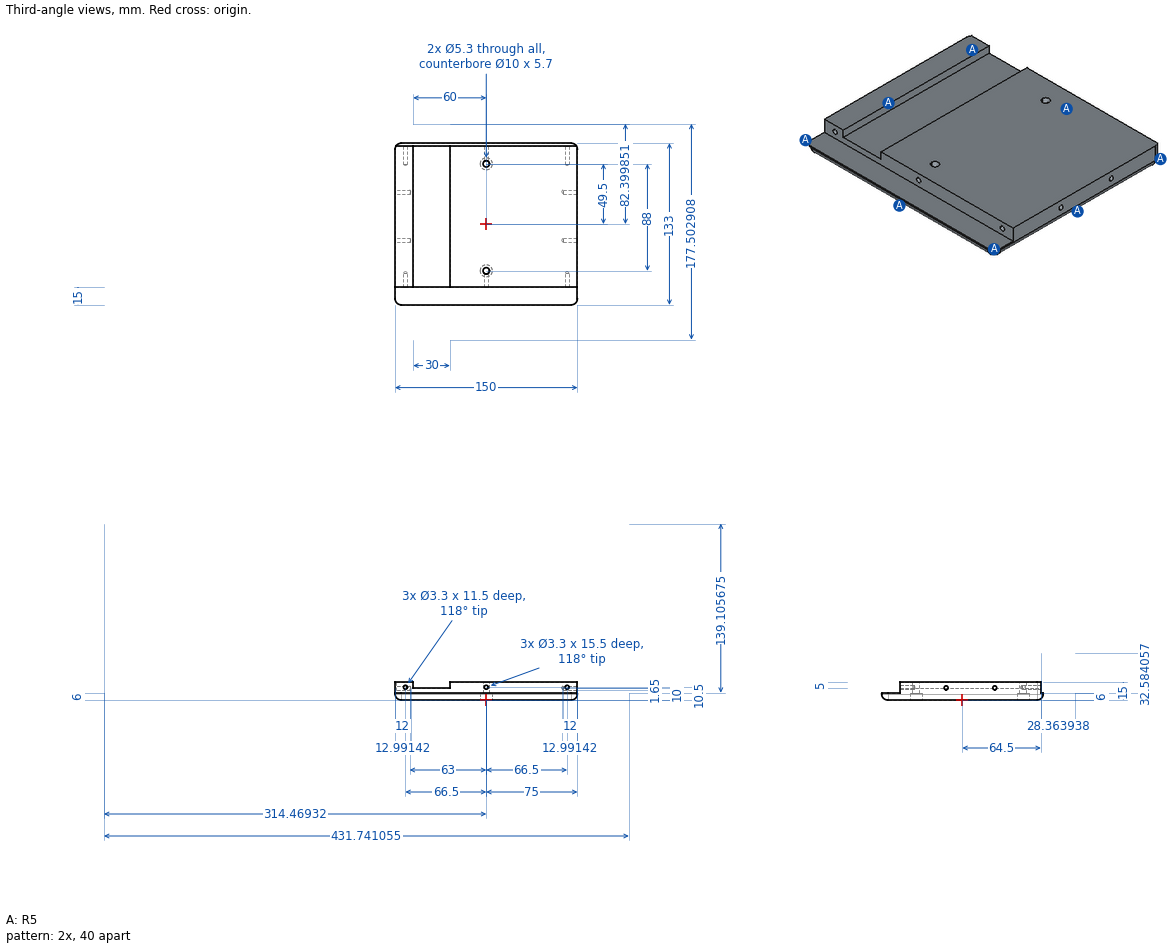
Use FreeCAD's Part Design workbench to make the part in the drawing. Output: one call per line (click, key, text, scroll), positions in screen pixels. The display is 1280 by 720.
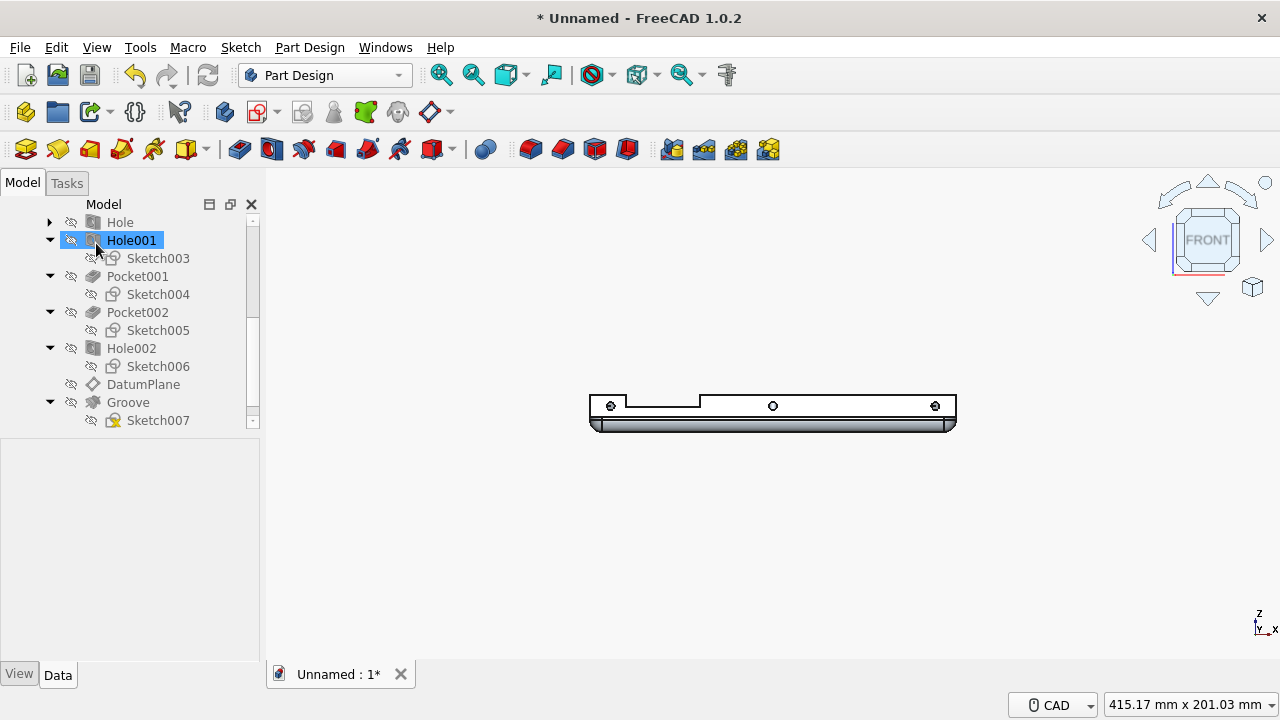
click(442, 76)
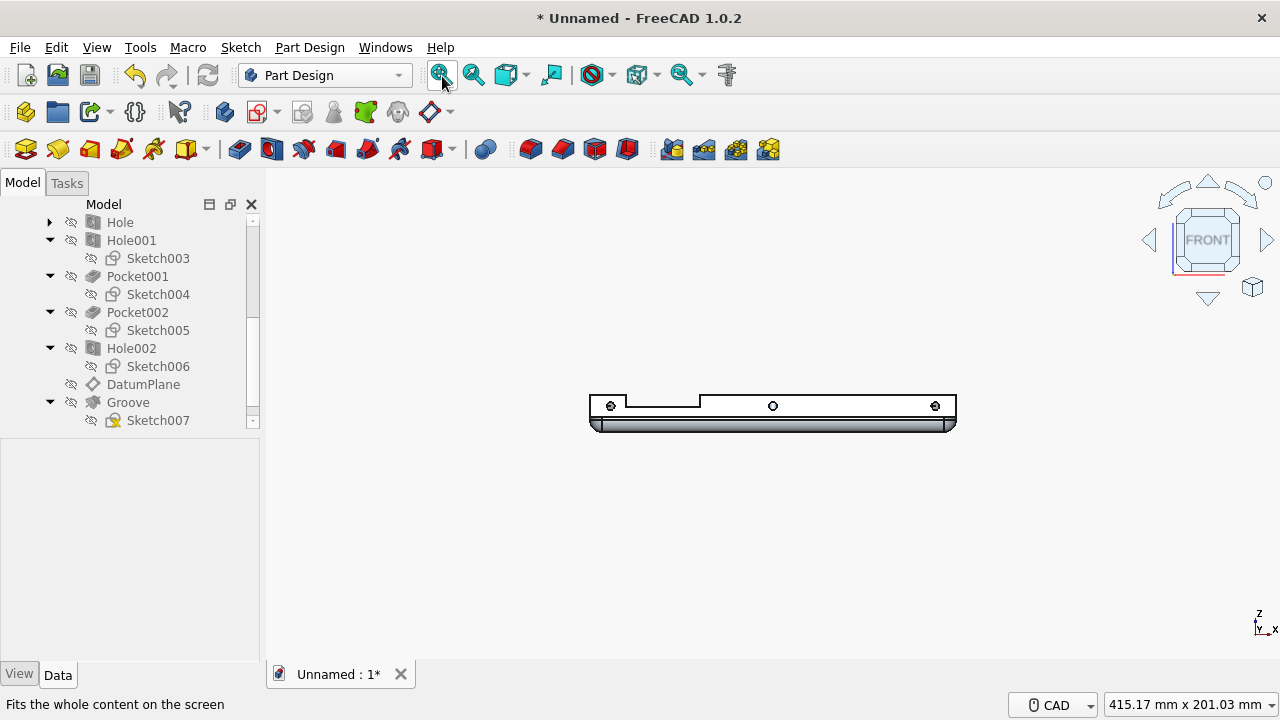
click(116, 402)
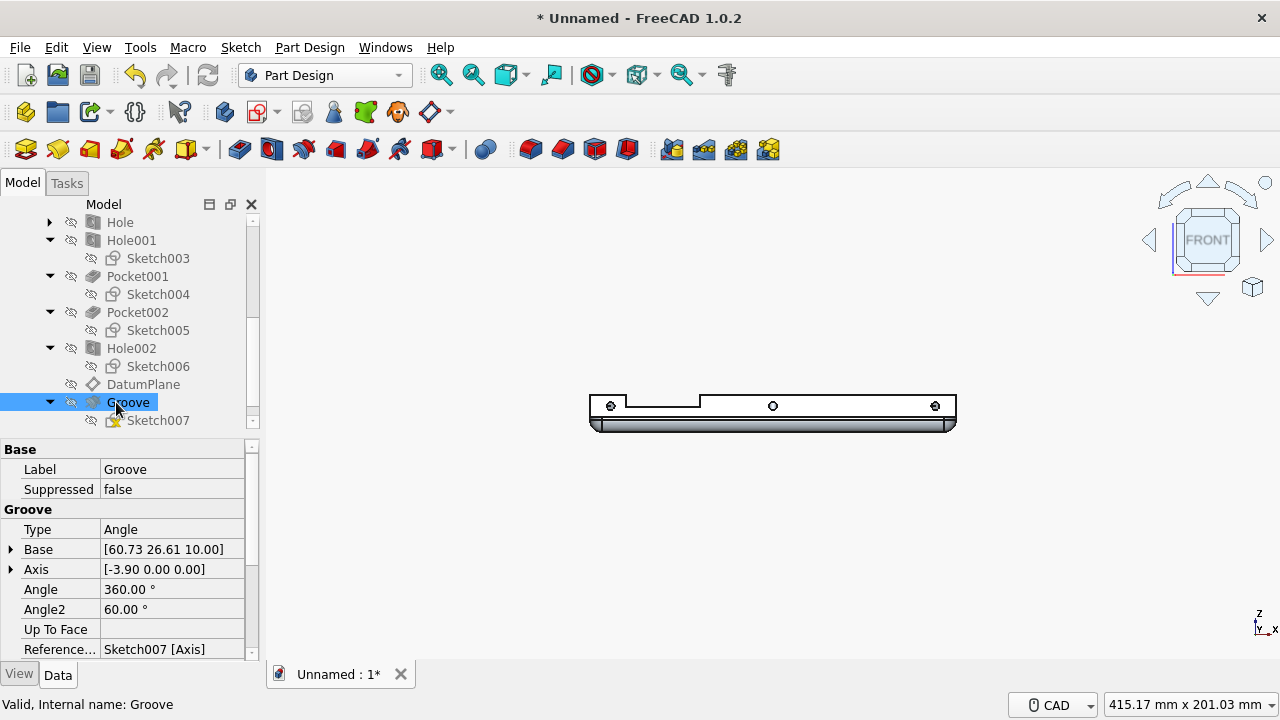
click(672, 150)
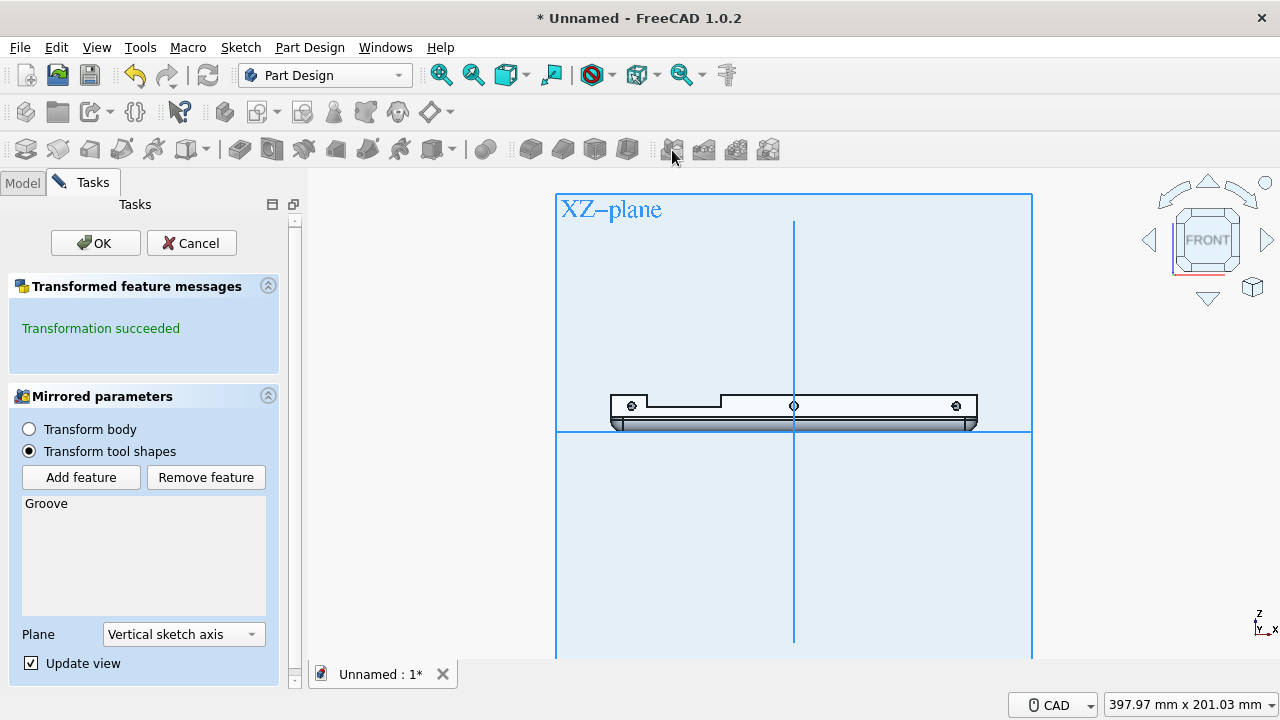
click(184, 634)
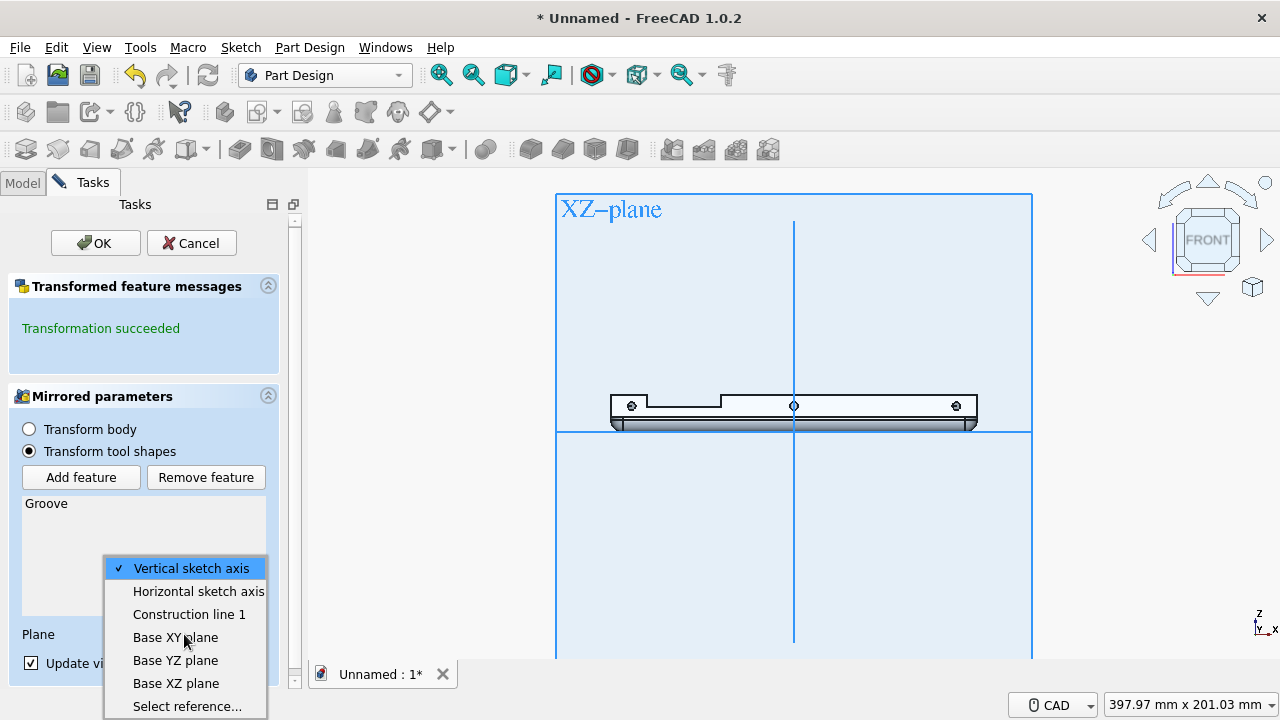
click(184, 660)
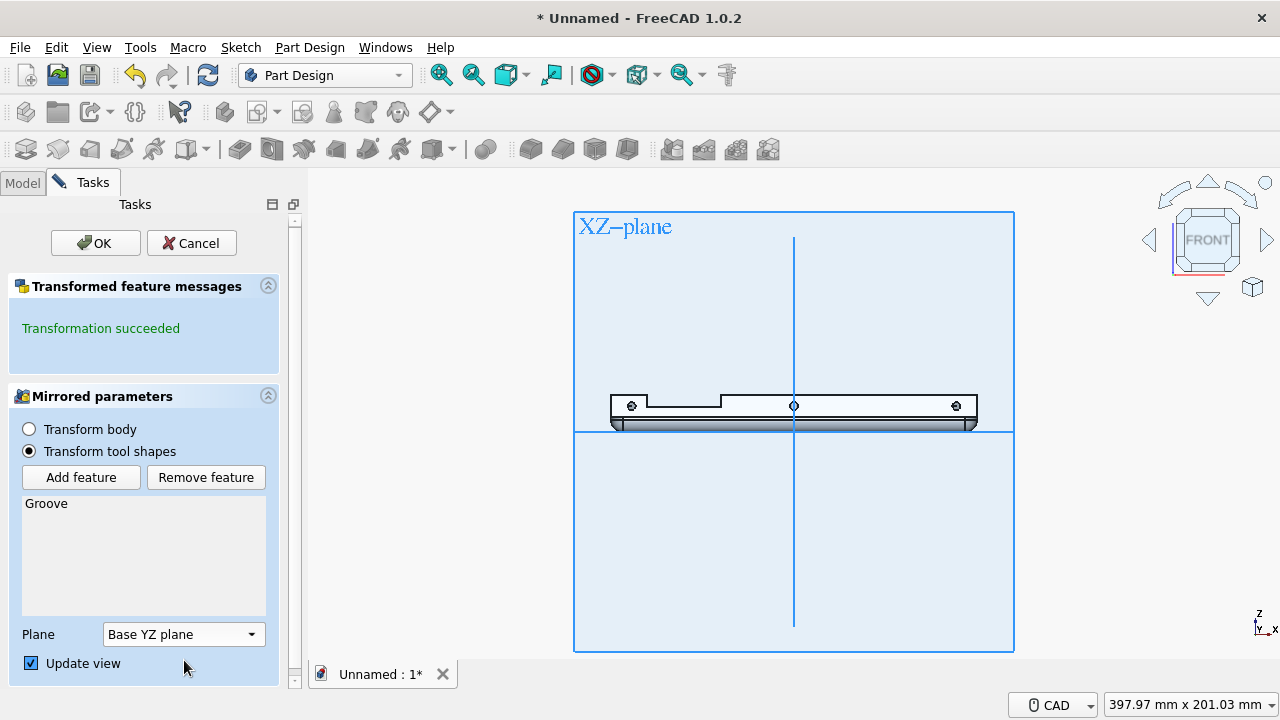
click(96, 243)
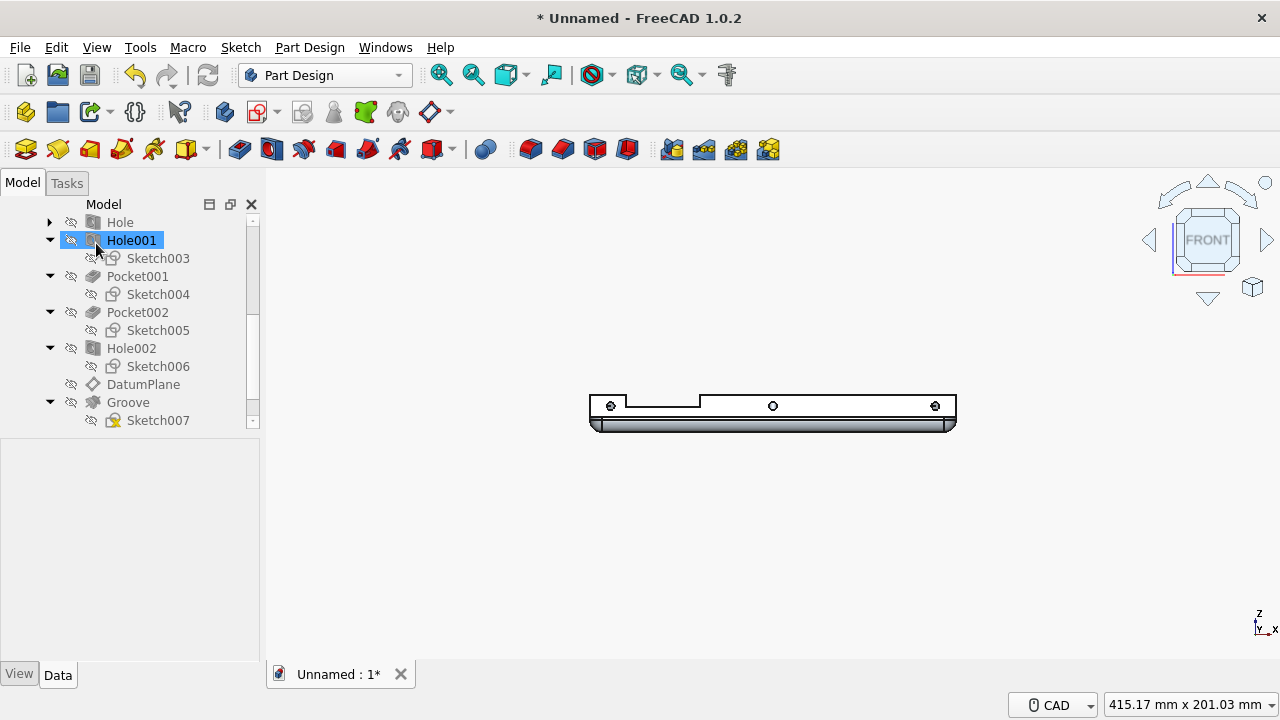
click(442, 76)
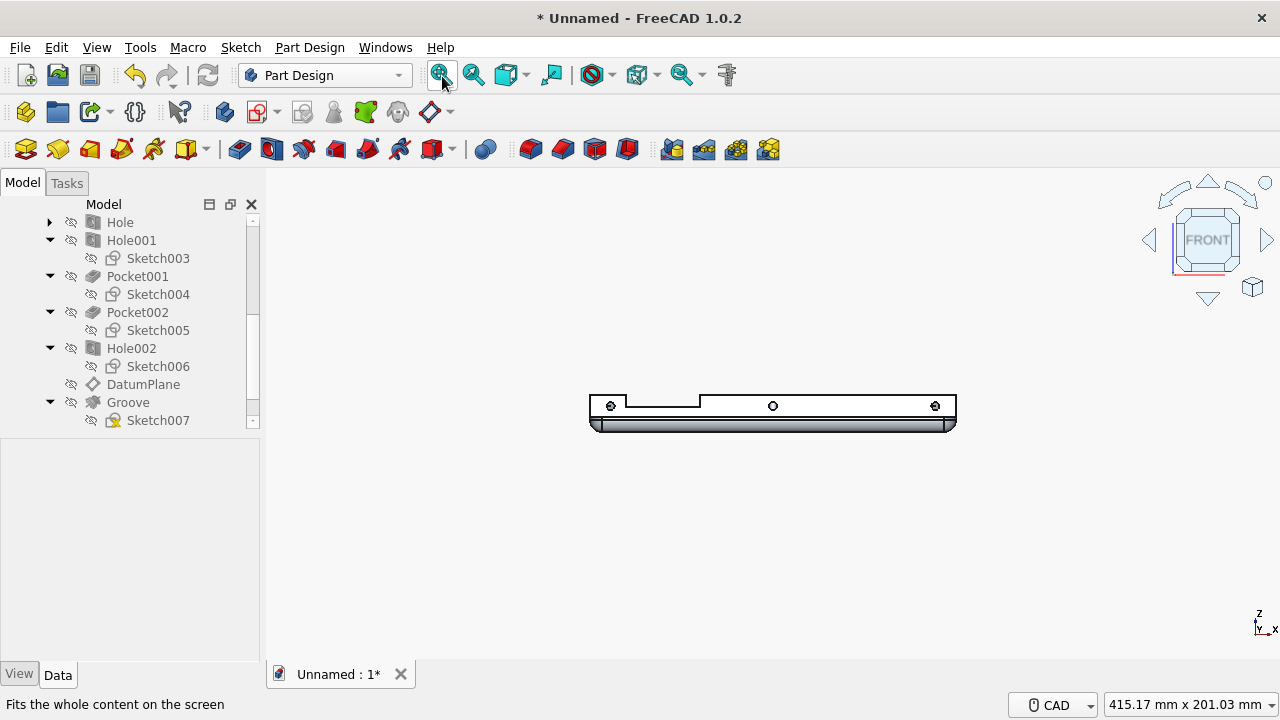
scroll(140, 326, down, 3)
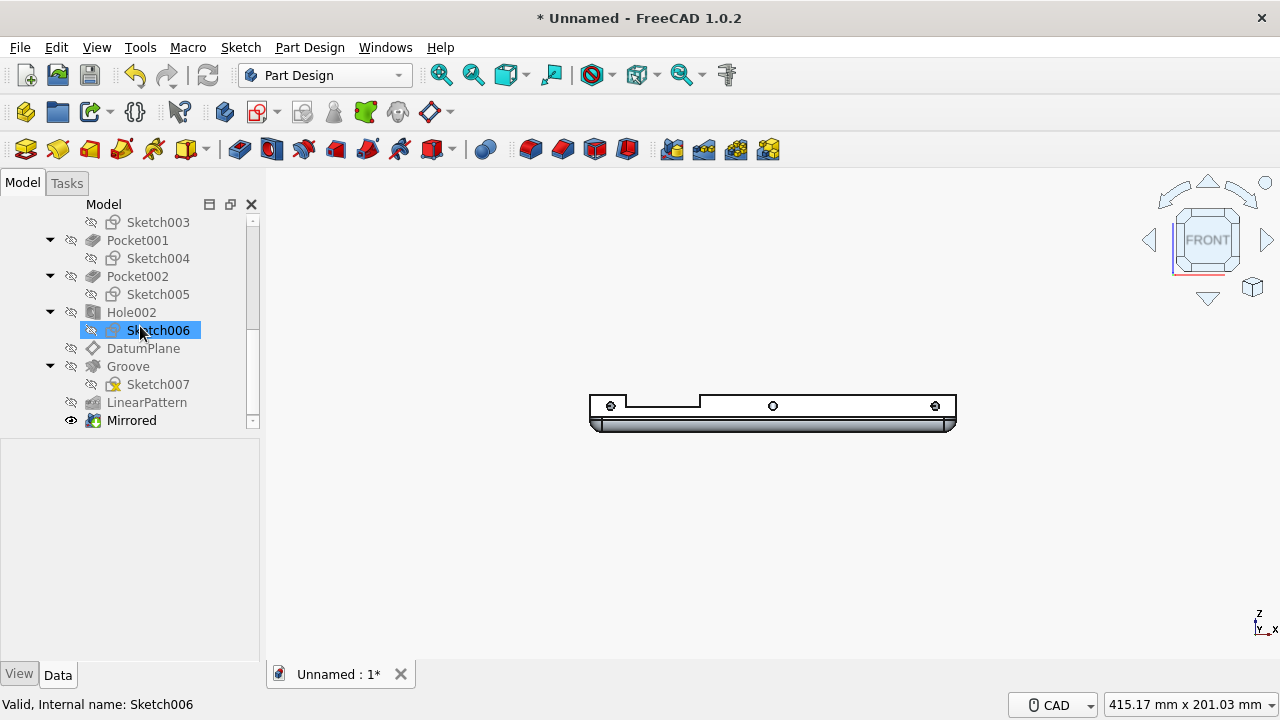
scroll(160, 326, up, 15)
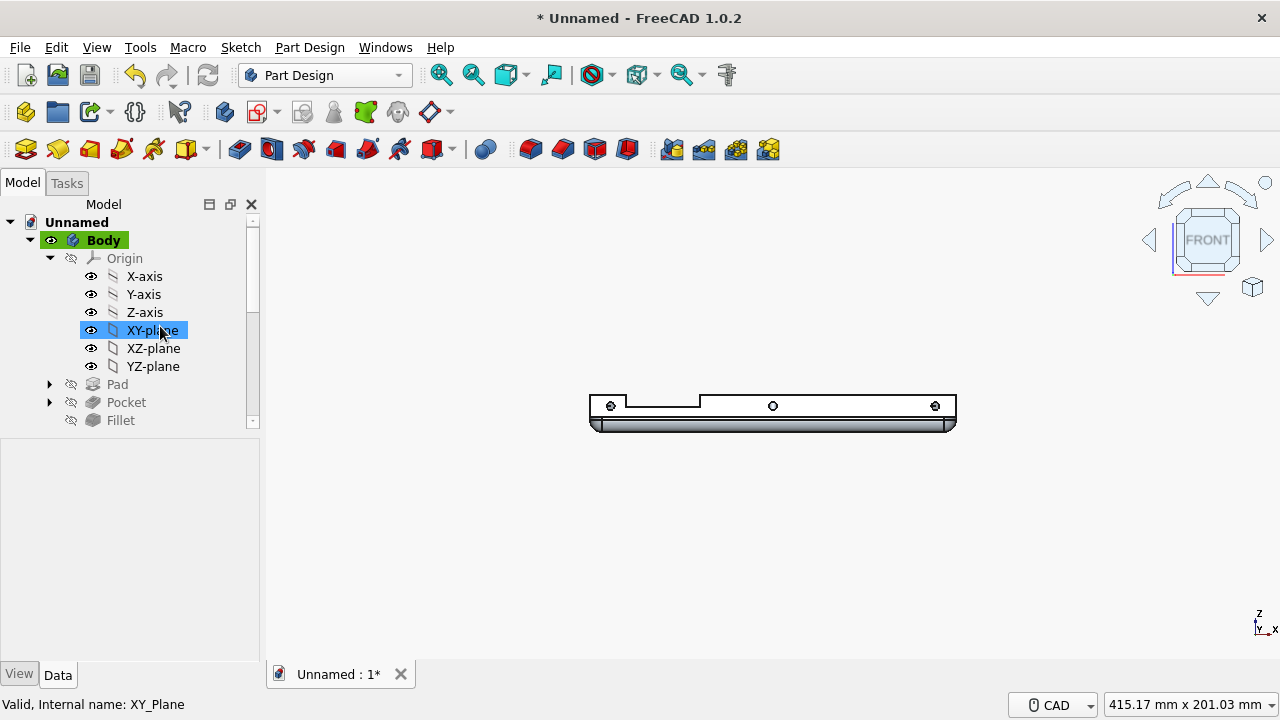
click(136, 348)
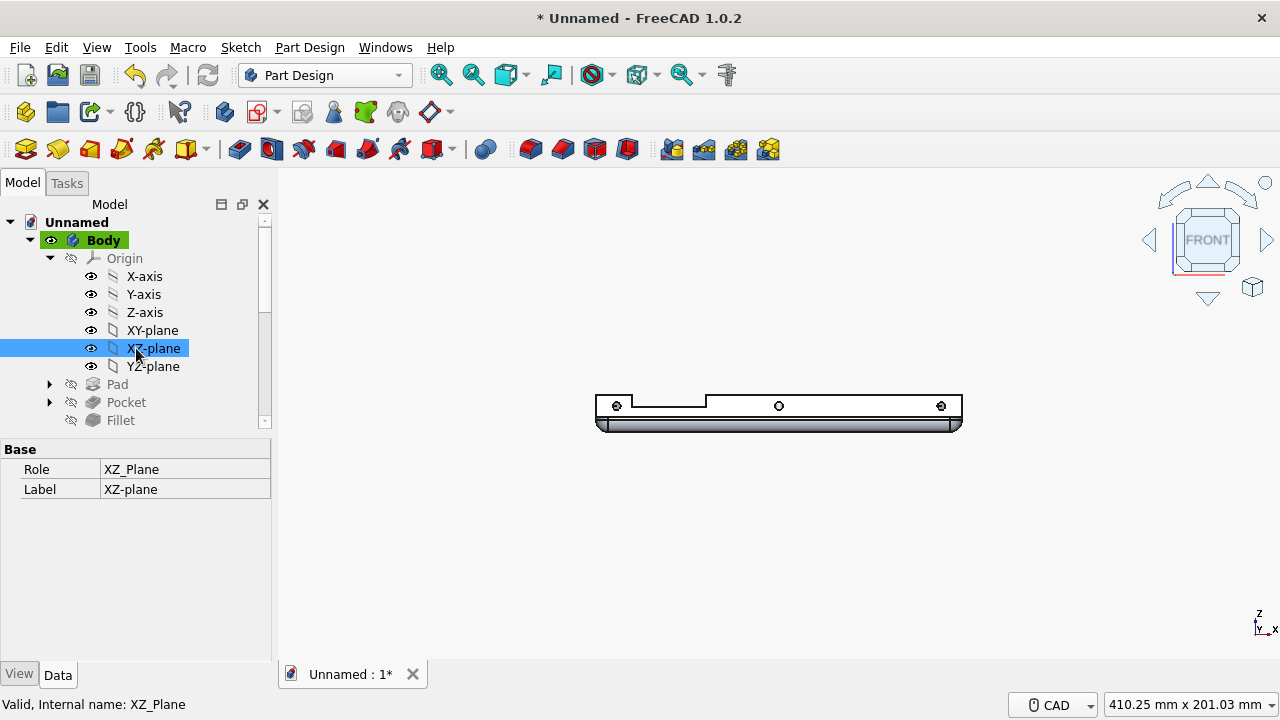
click(430, 112)